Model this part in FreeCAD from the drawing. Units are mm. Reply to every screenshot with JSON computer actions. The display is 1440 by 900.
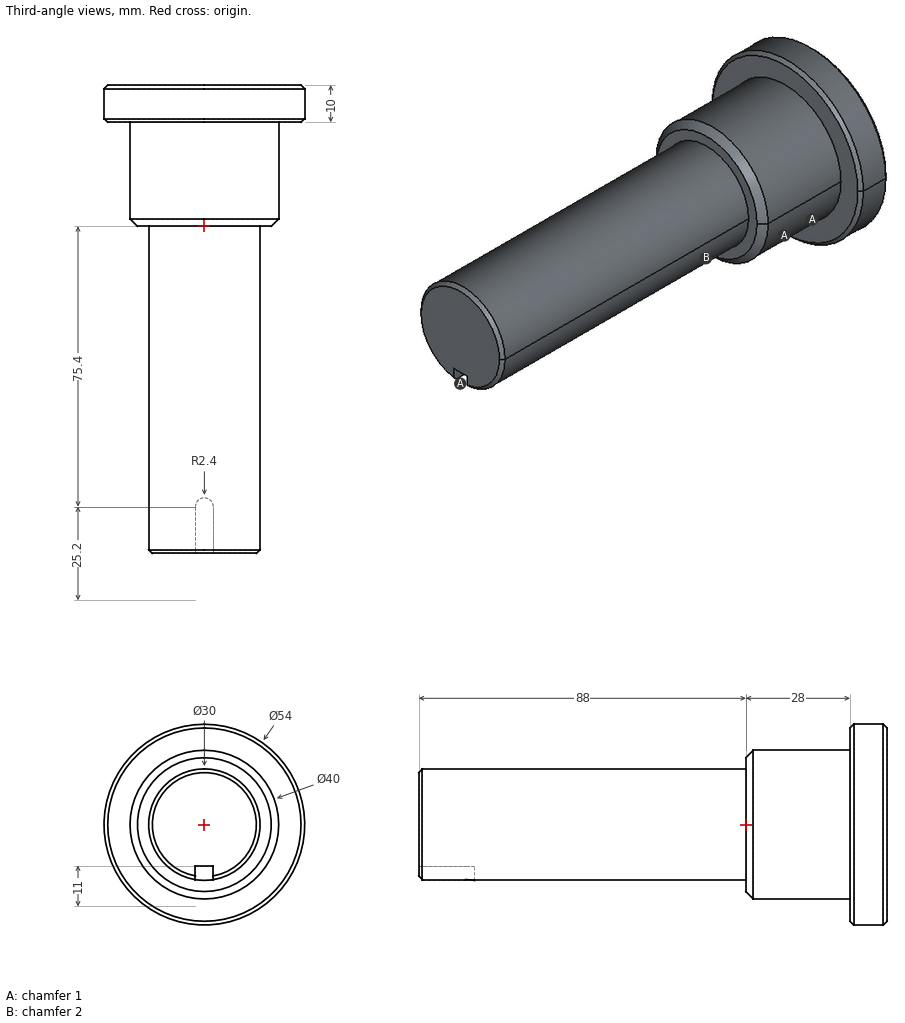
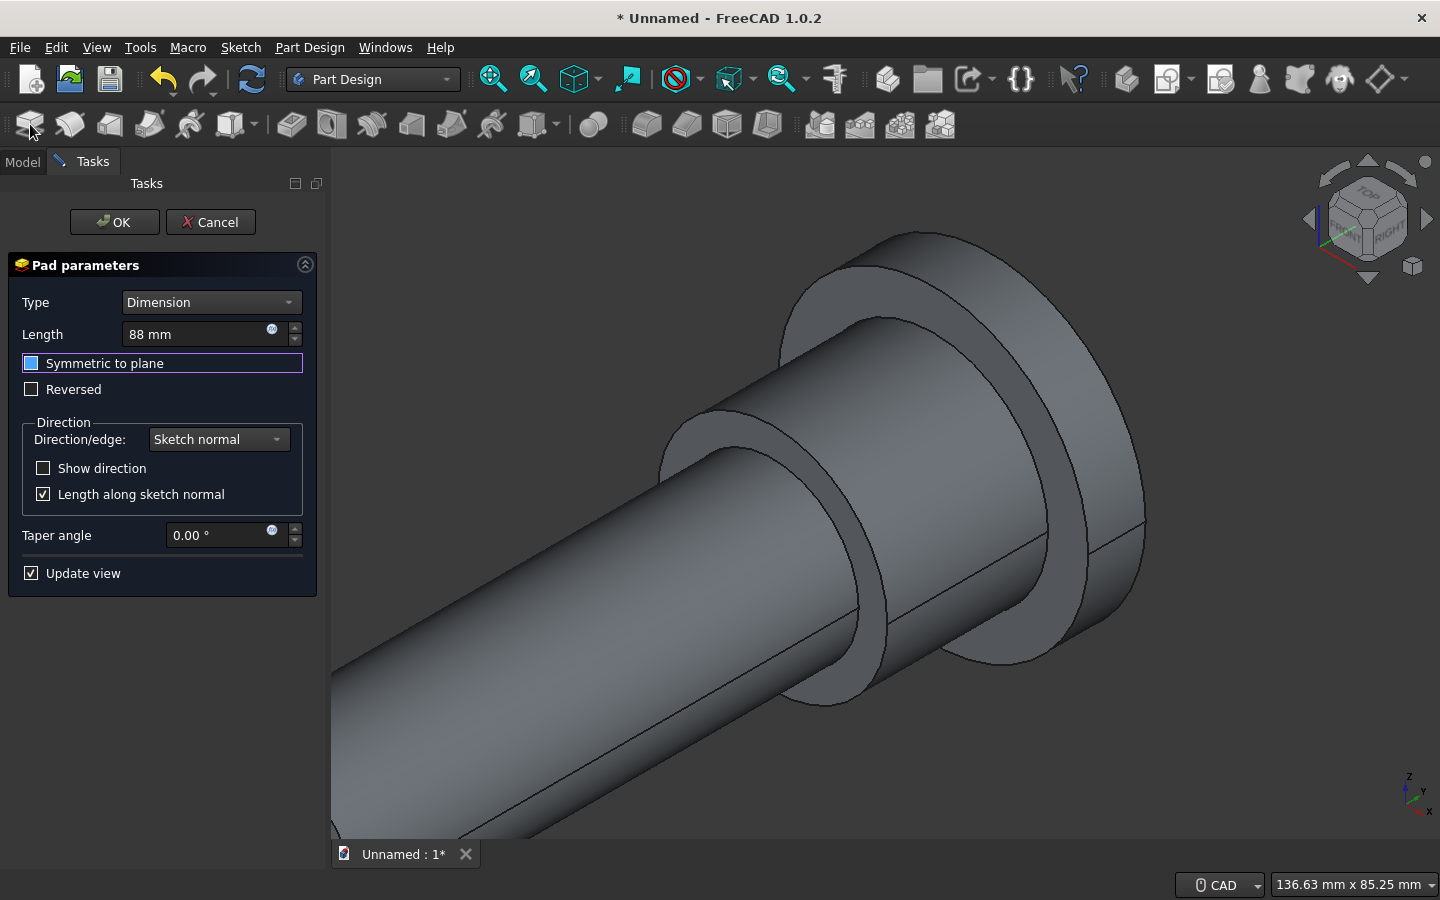
{"action": "left_click", "coordinate": [115, 222]}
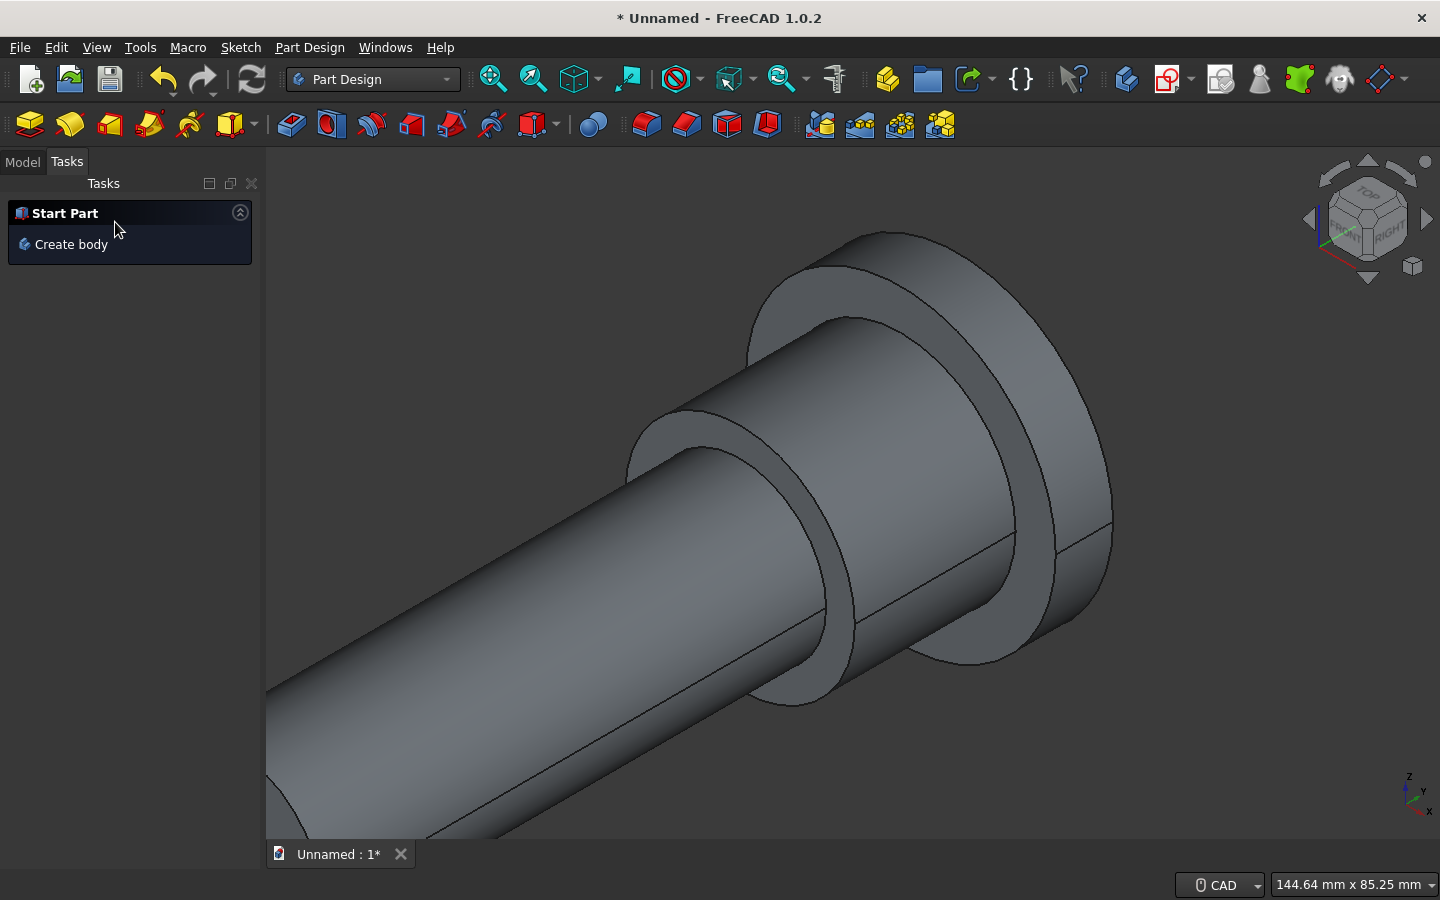
{"action": "key", "text": "v f"}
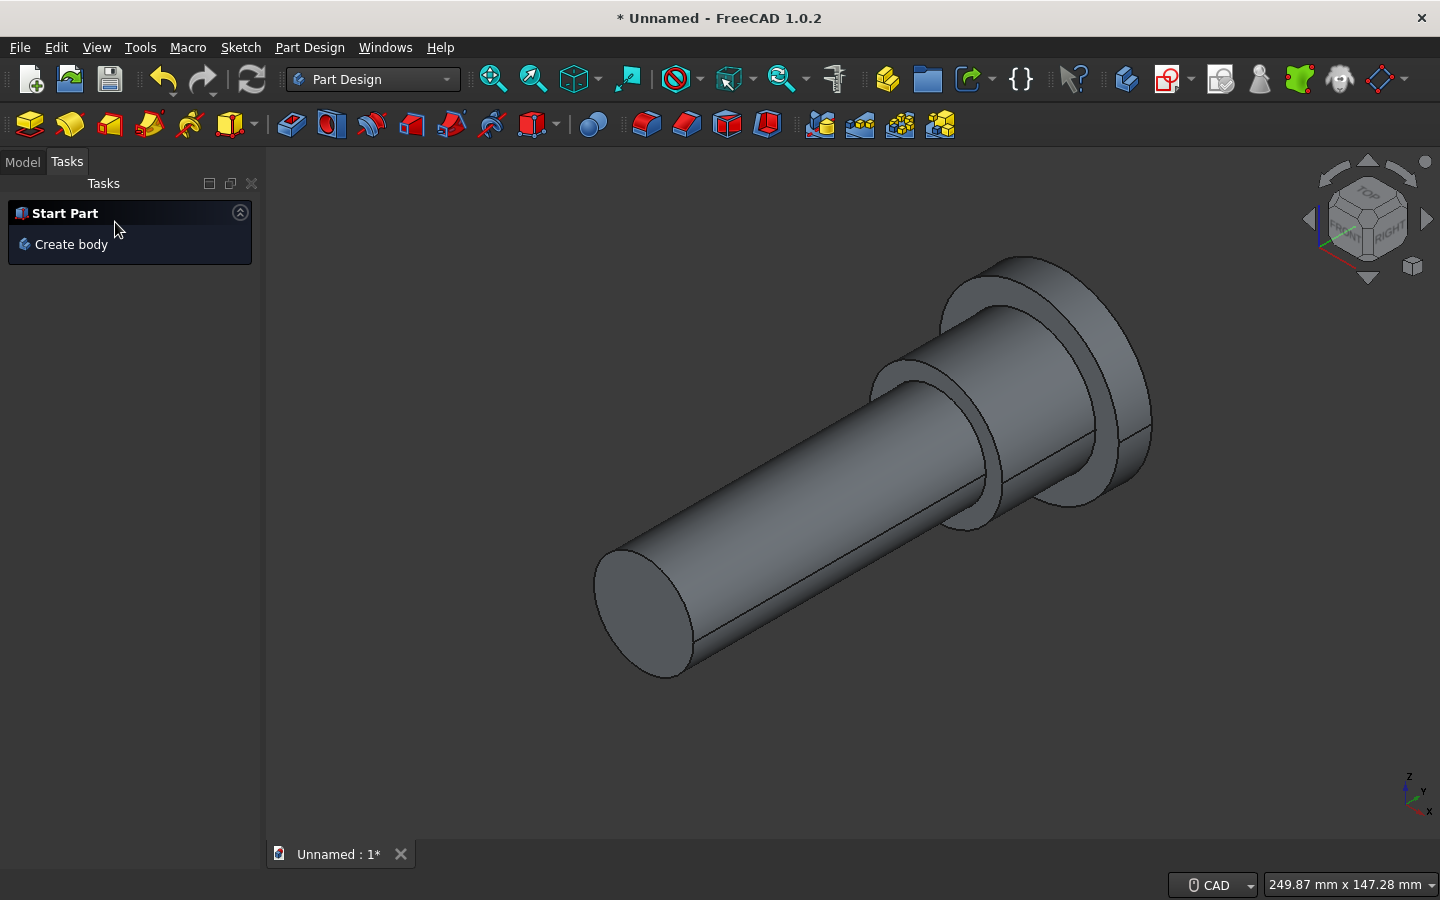
{"action": "left_click", "coordinate": [628, 549]}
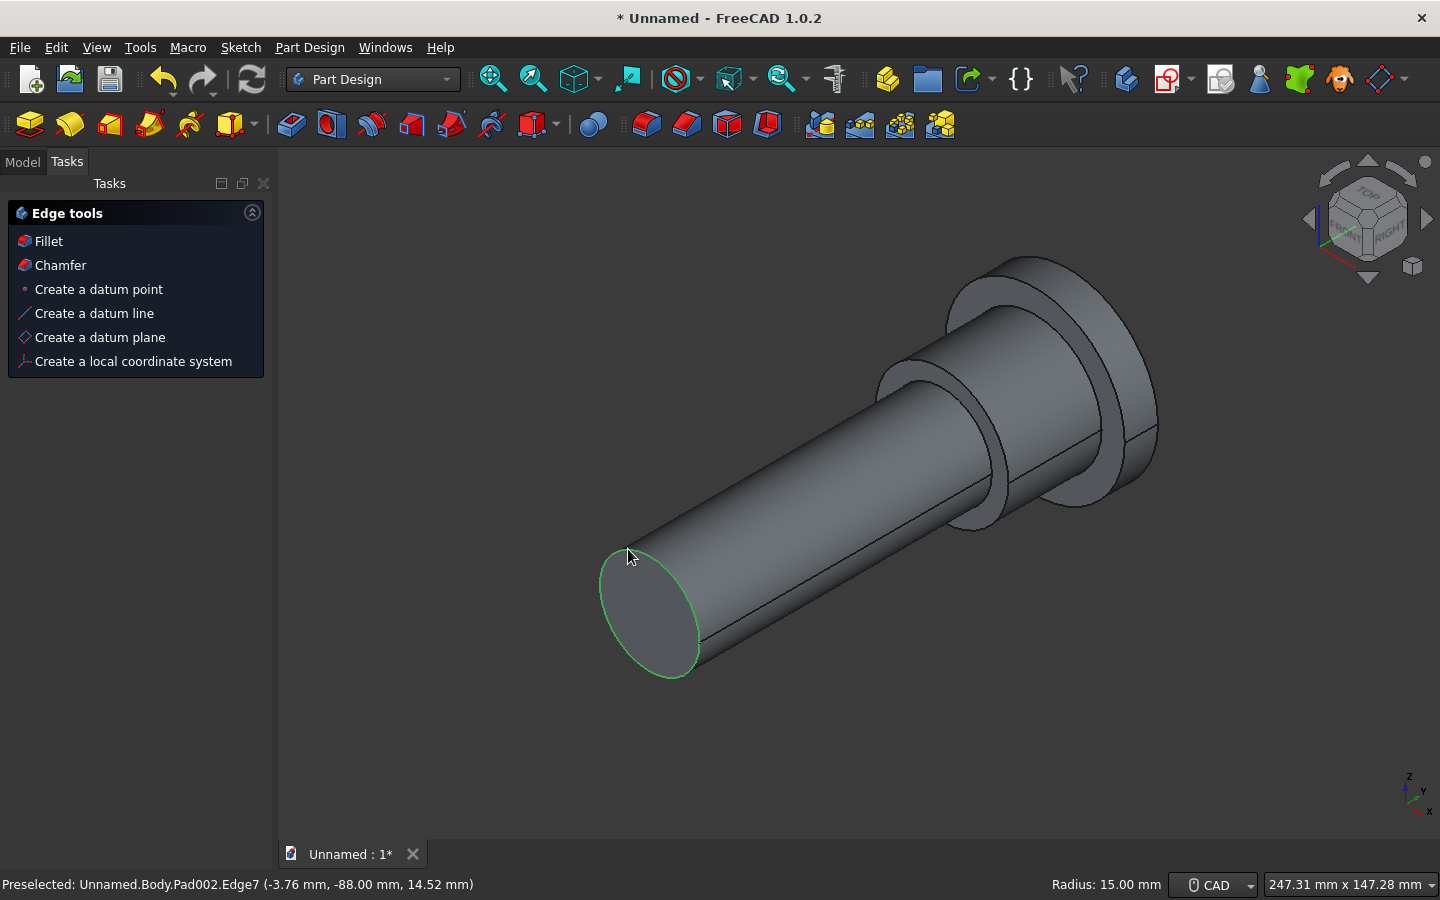
{"action": "left_click", "coordinate": [1007, 276], "text": "ctrl"}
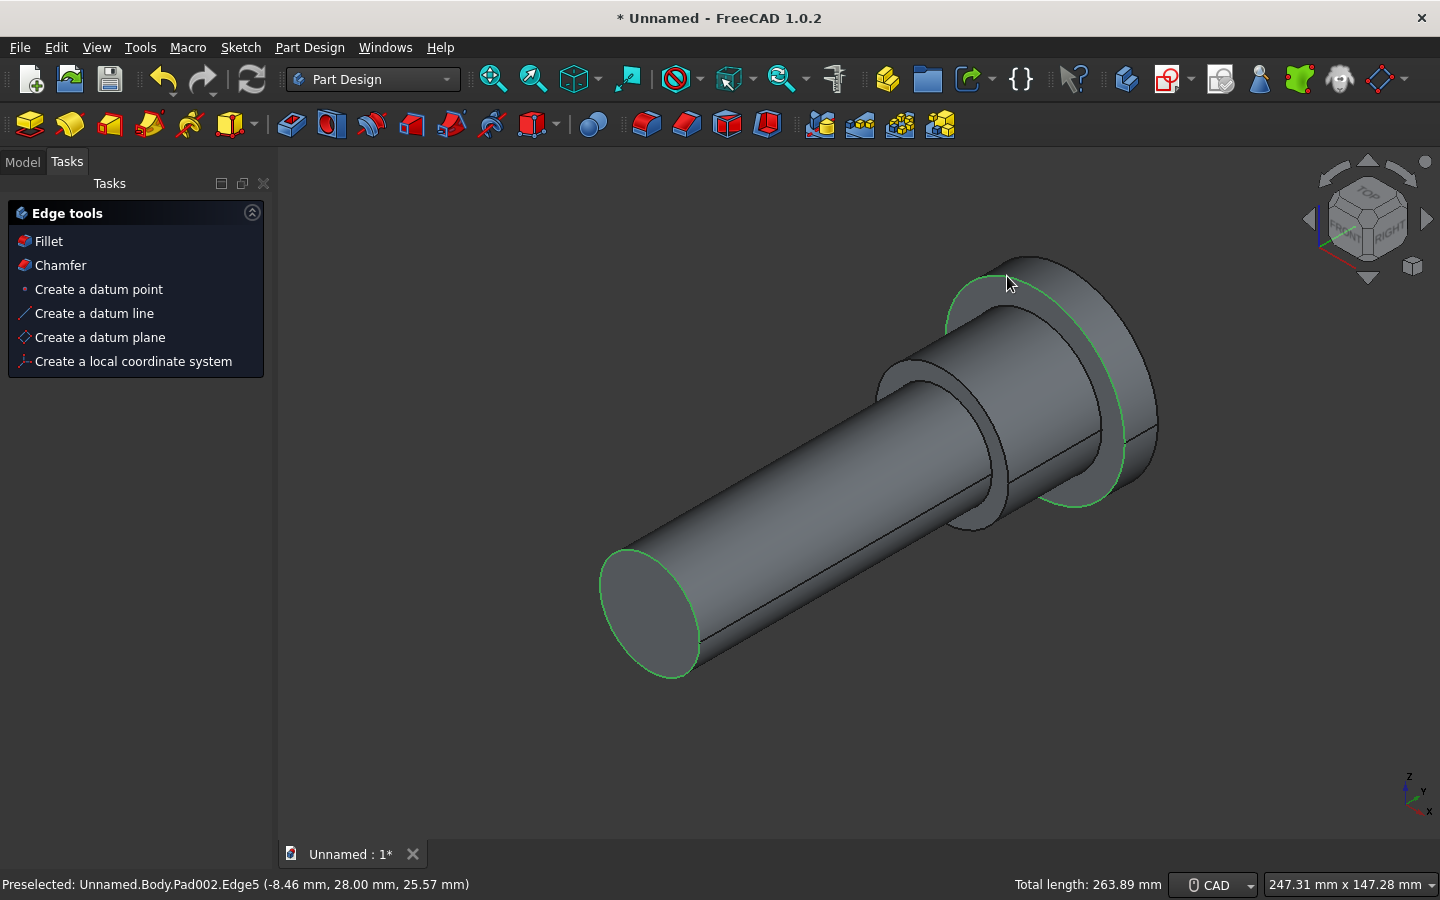
{"action": "key", "text": "2"}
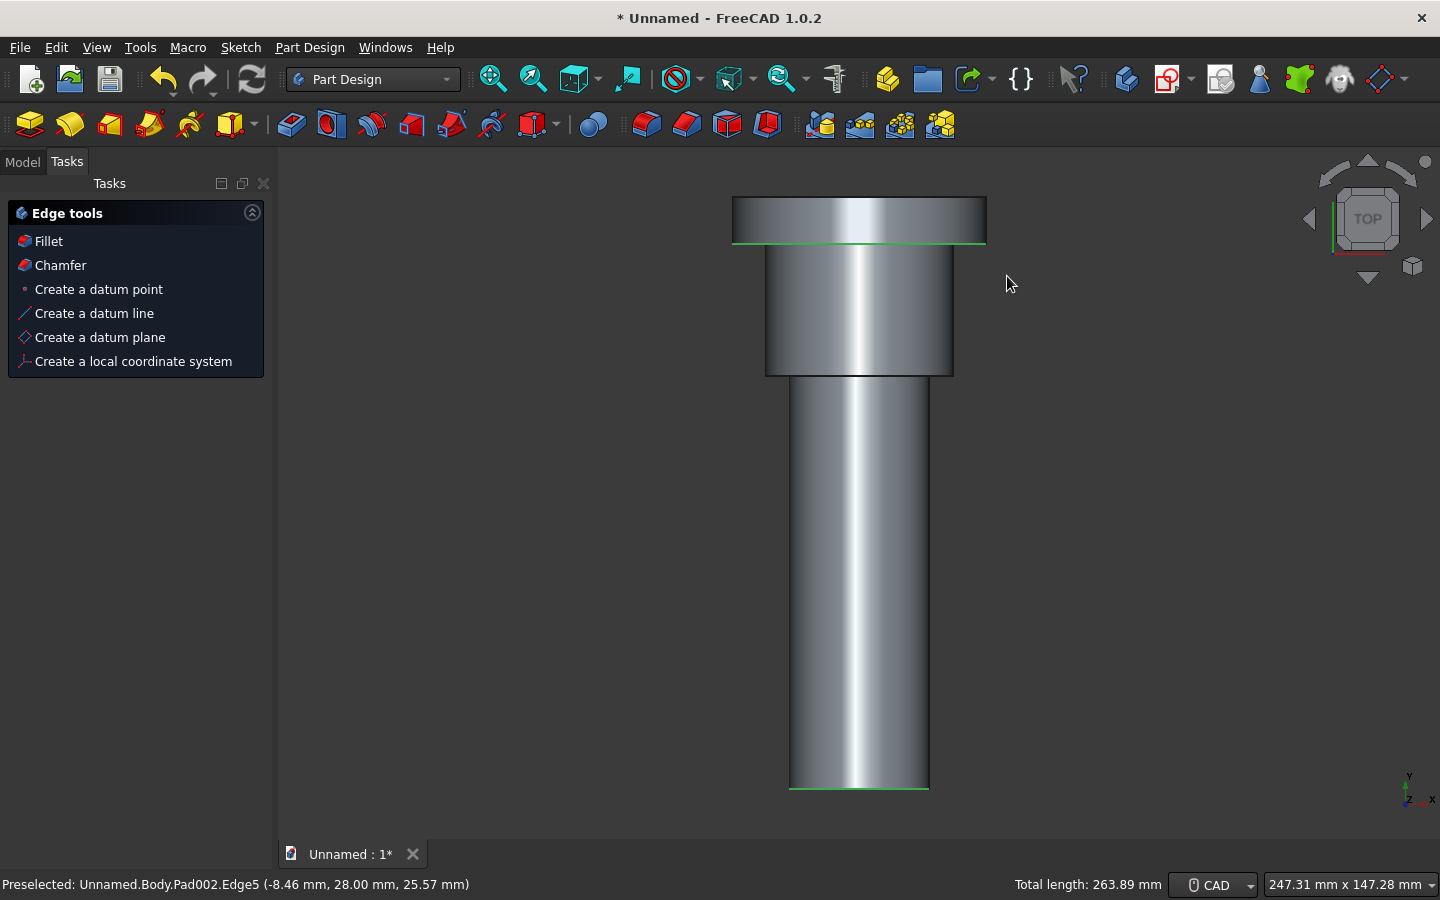
{"action": "left_click", "coordinate": [756, 196], "text": "ctrl"}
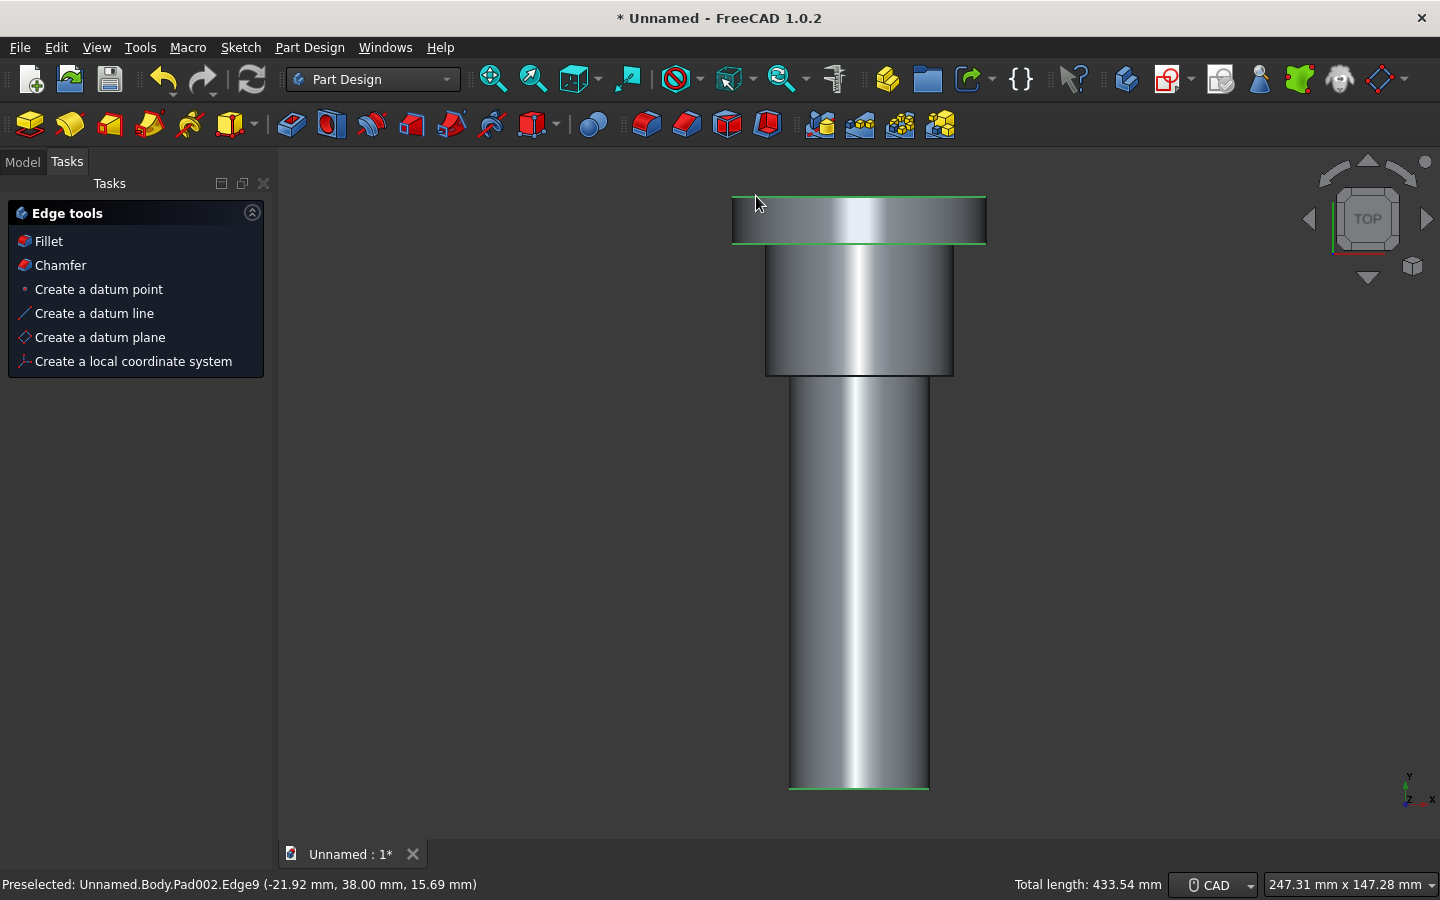
{"action": "left_click", "coordinate": [688, 124]}